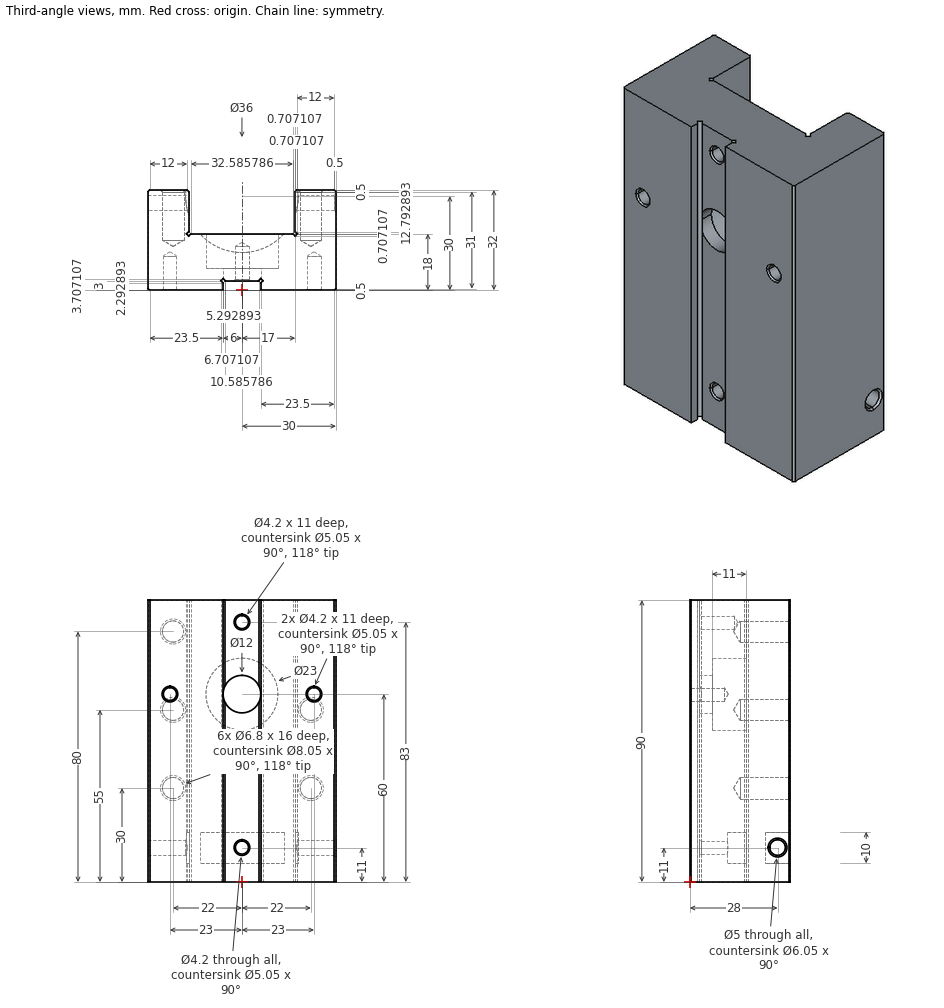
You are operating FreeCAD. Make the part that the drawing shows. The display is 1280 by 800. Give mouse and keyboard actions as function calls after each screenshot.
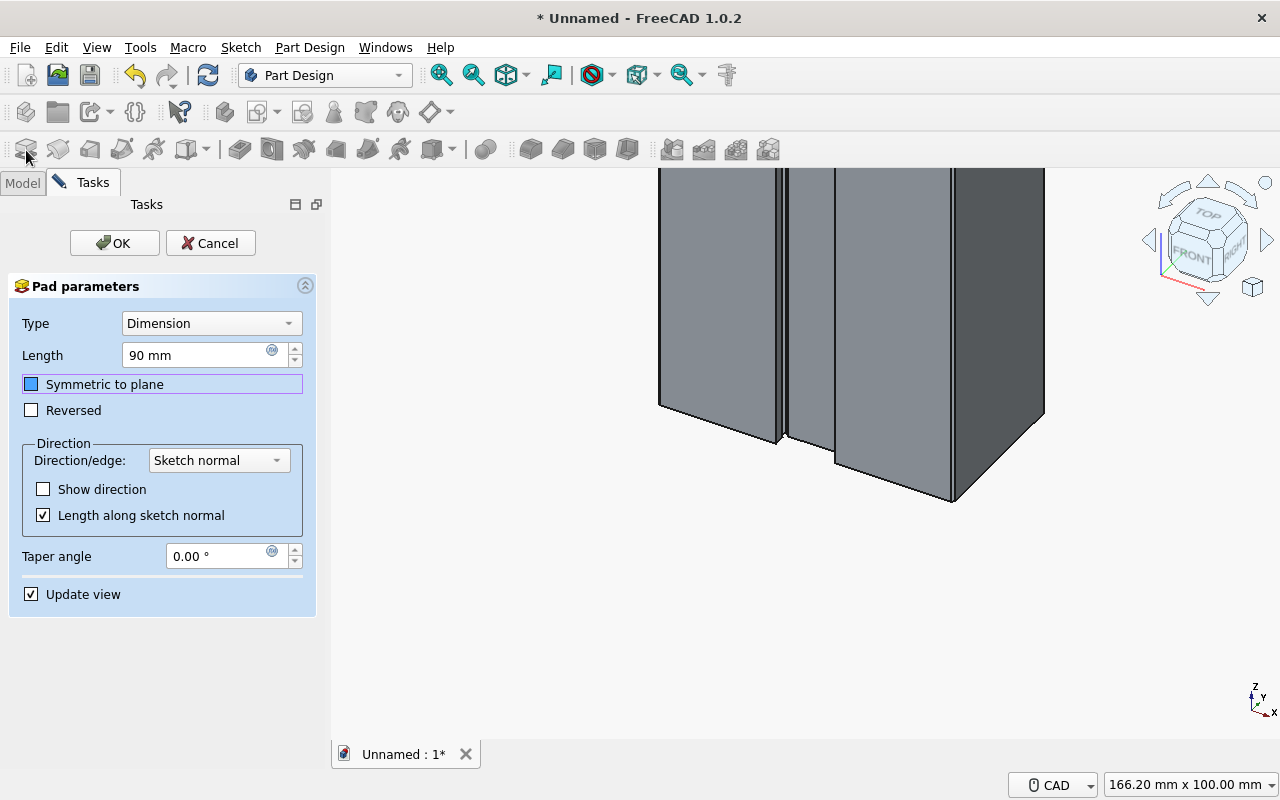
click(115, 243)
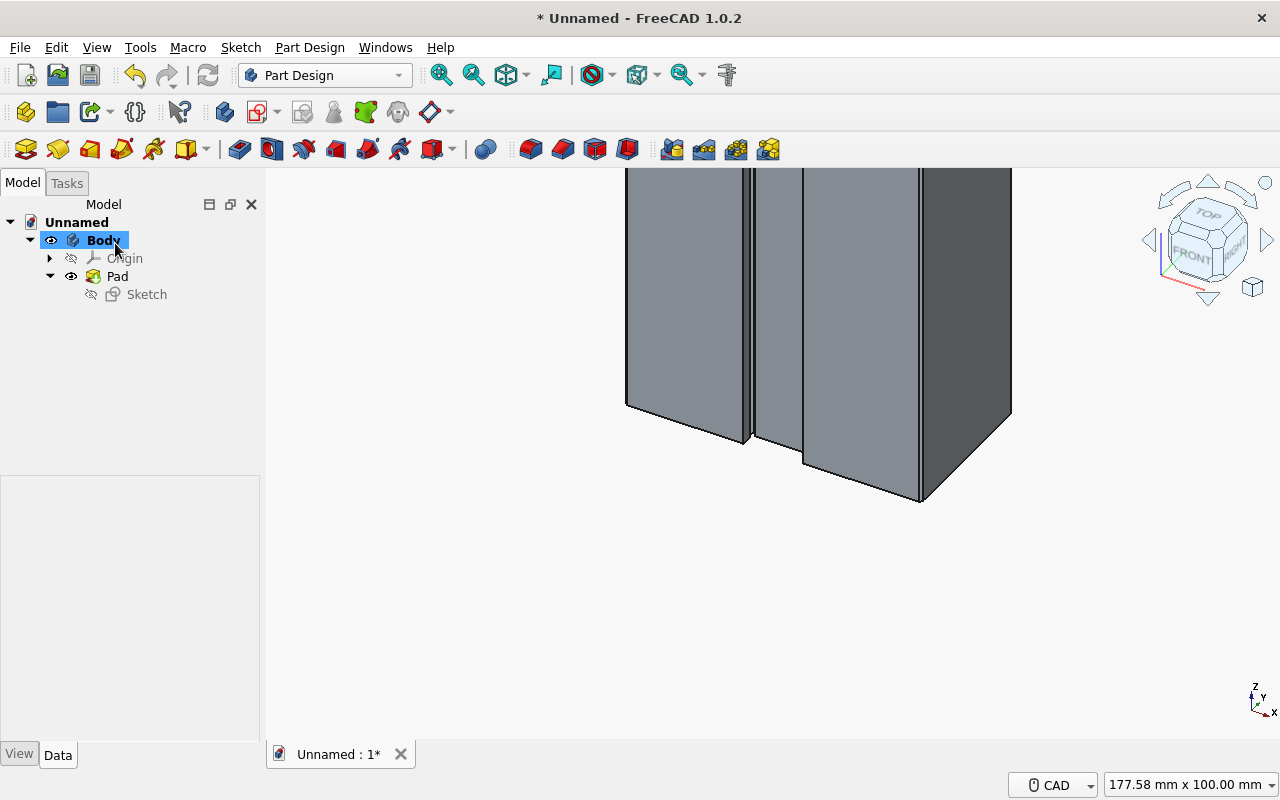
click(442, 76)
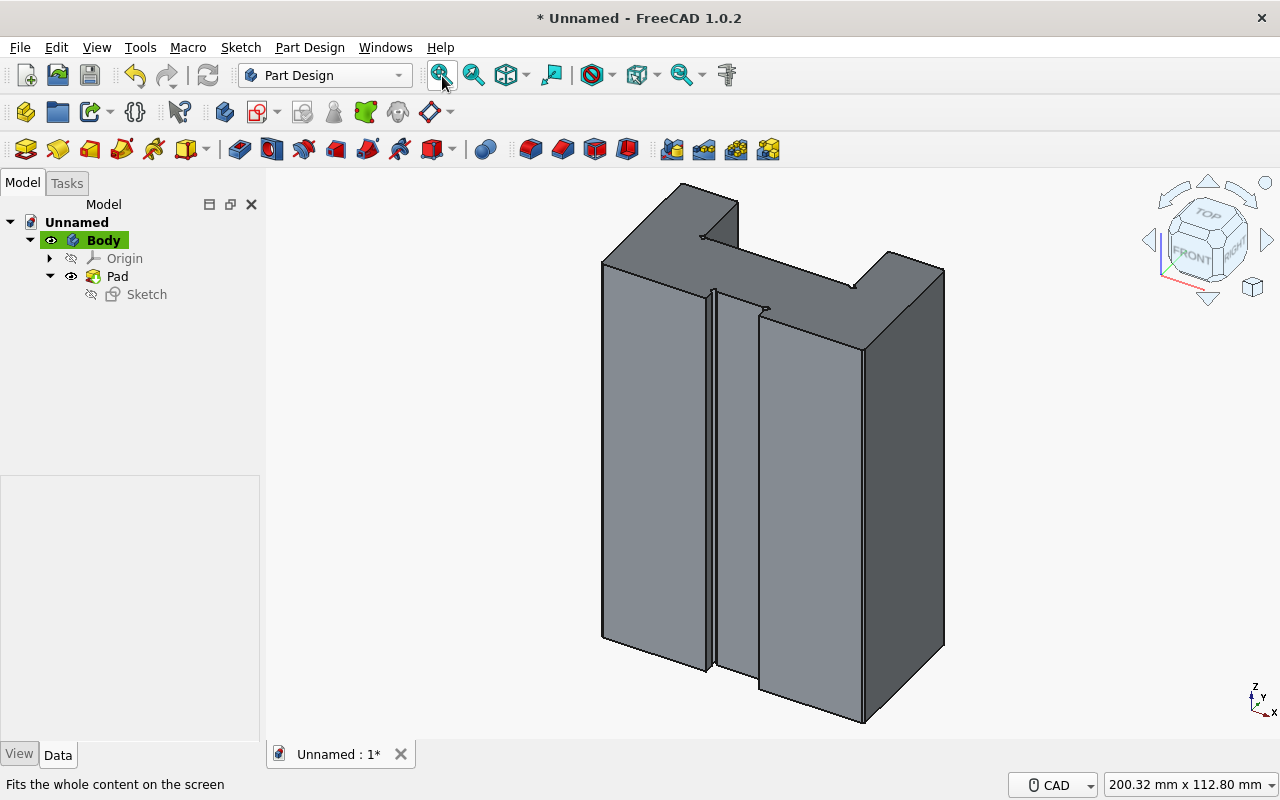
key(4)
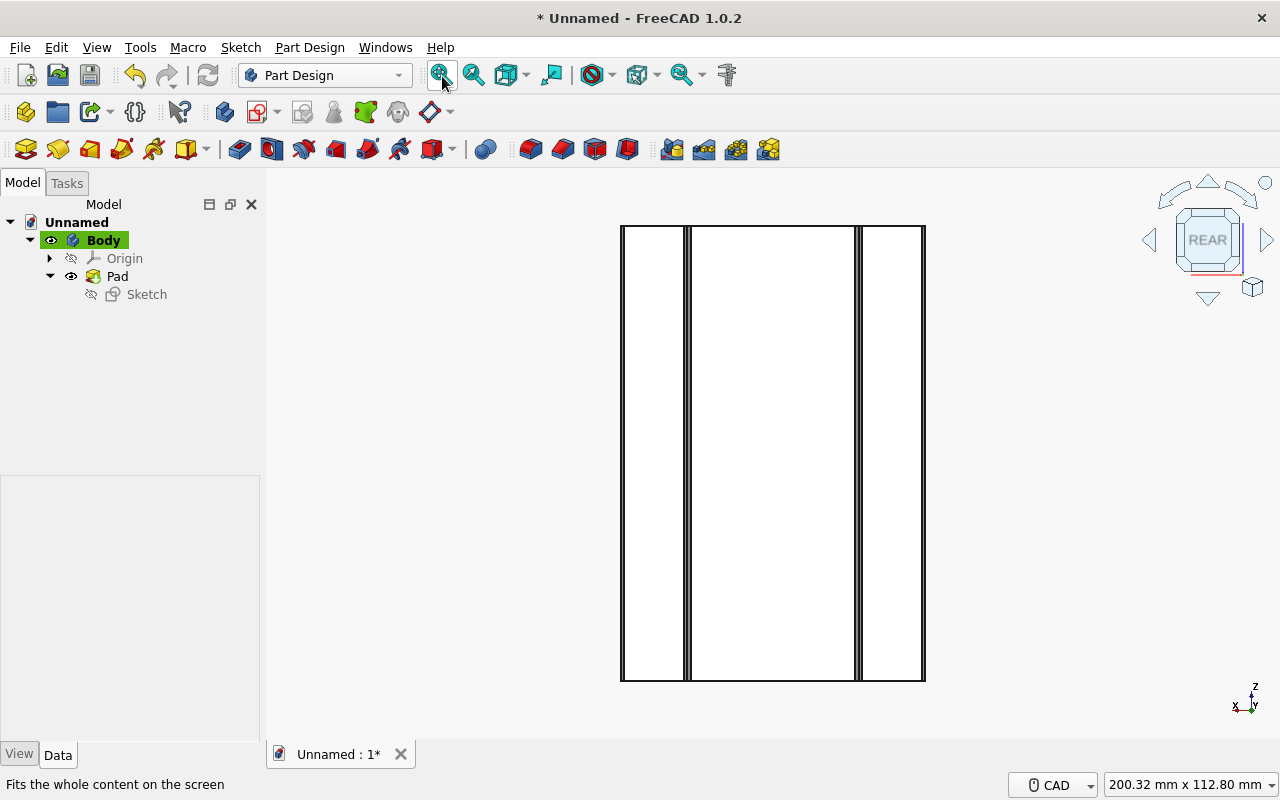
click(773, 322)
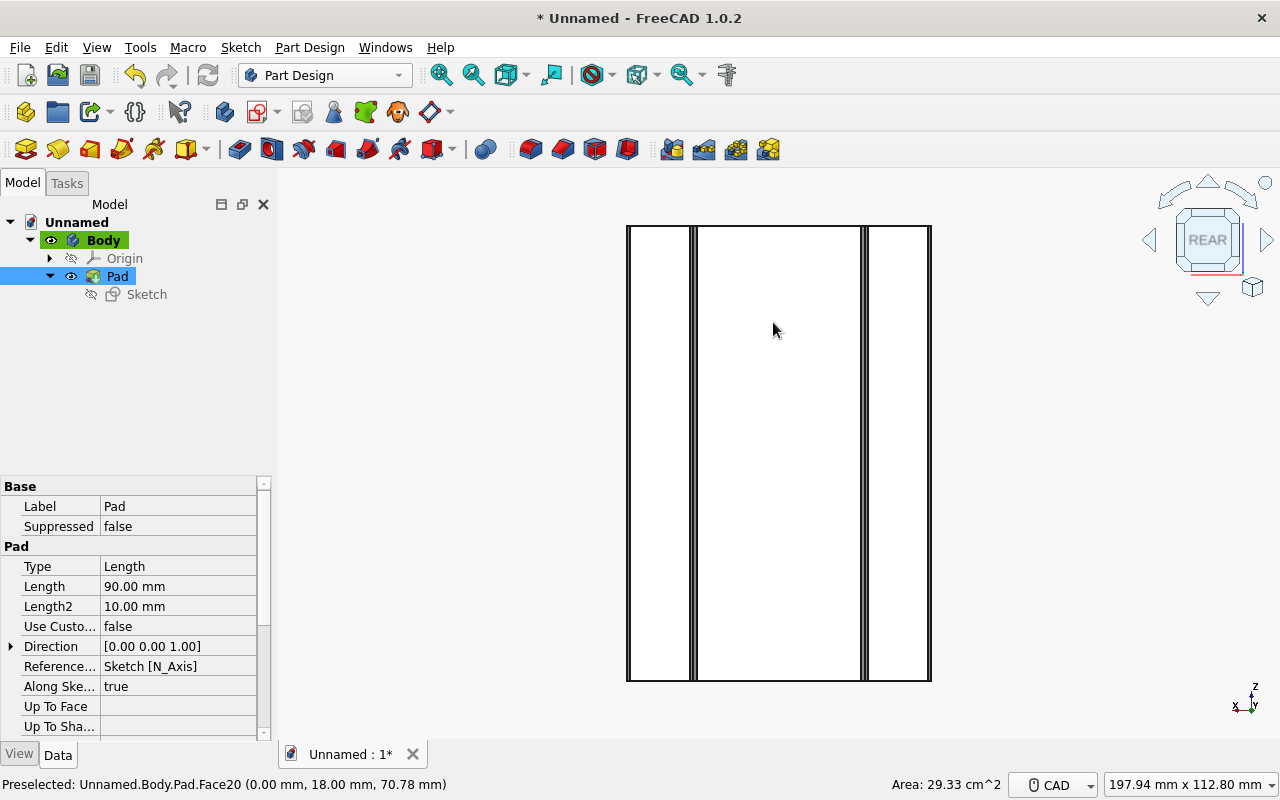
click(258, 112)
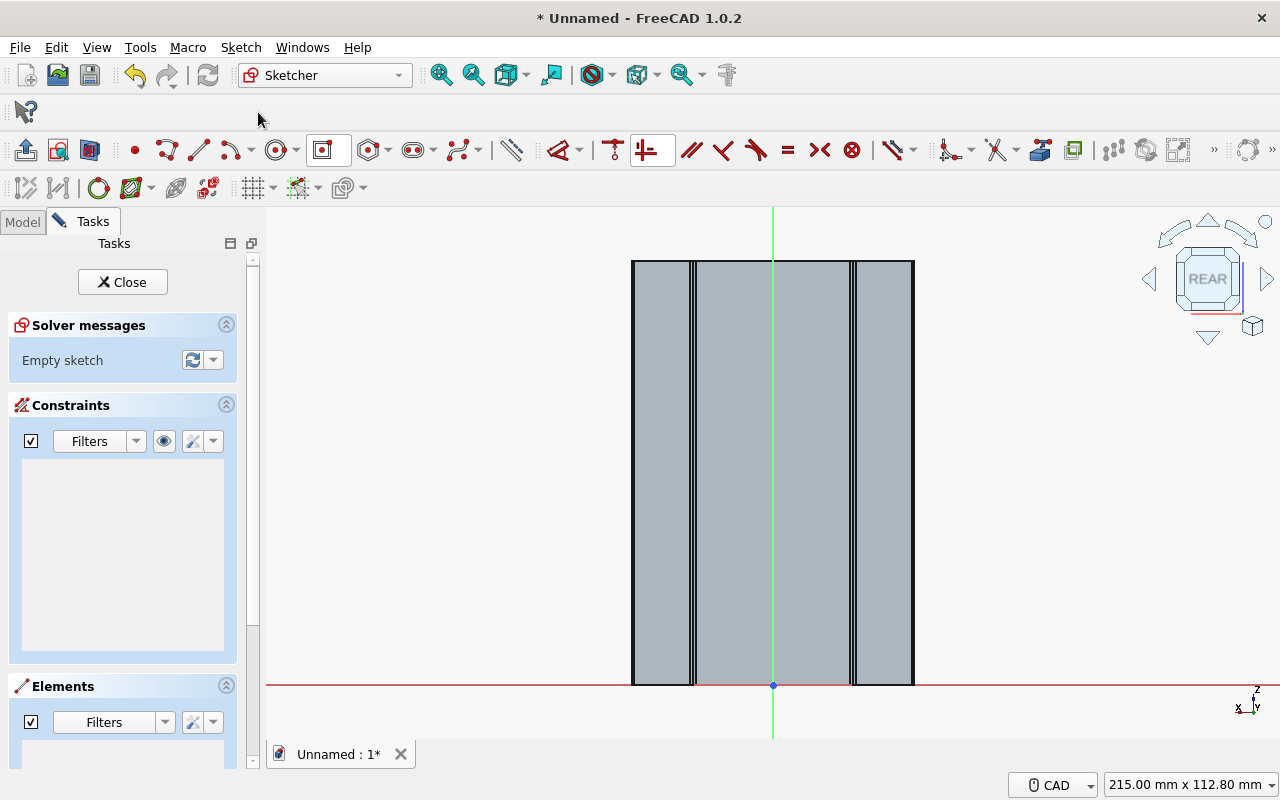
click(90, 150)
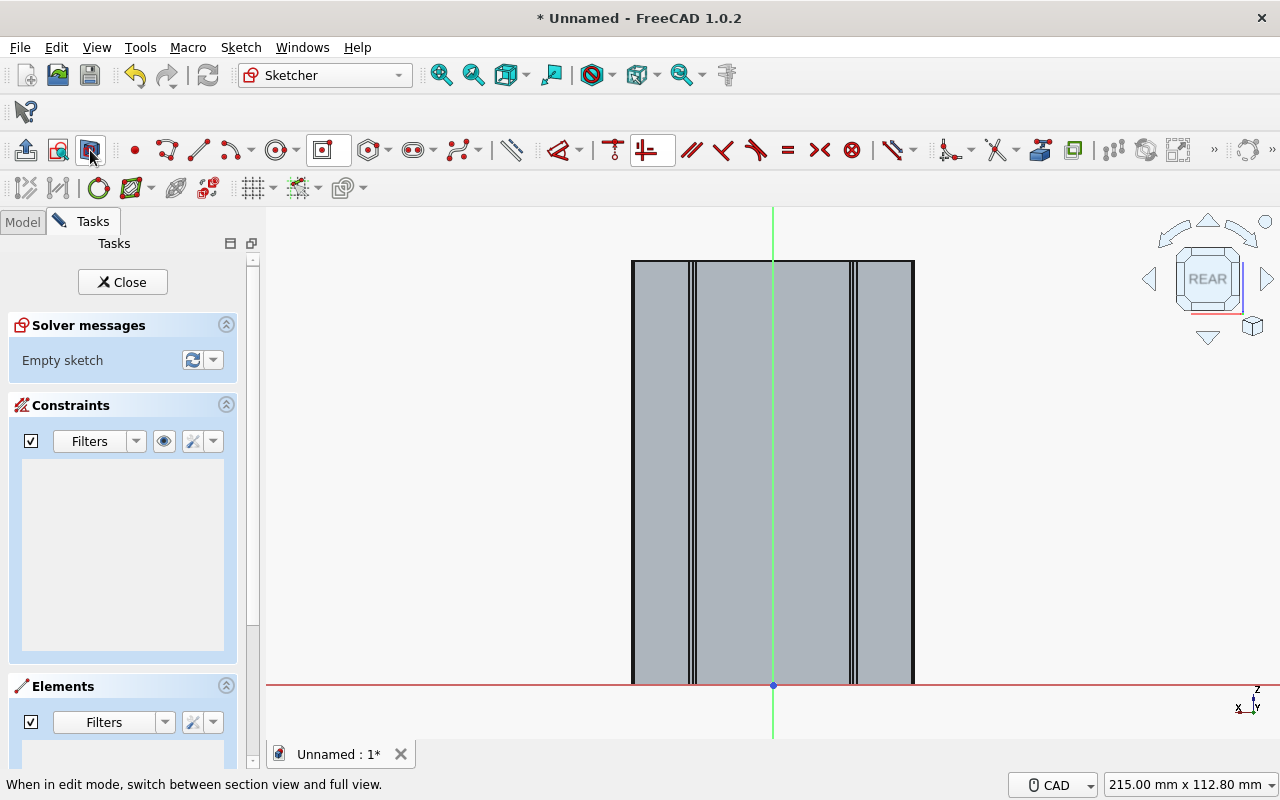
scroll(803, 372, up, 6)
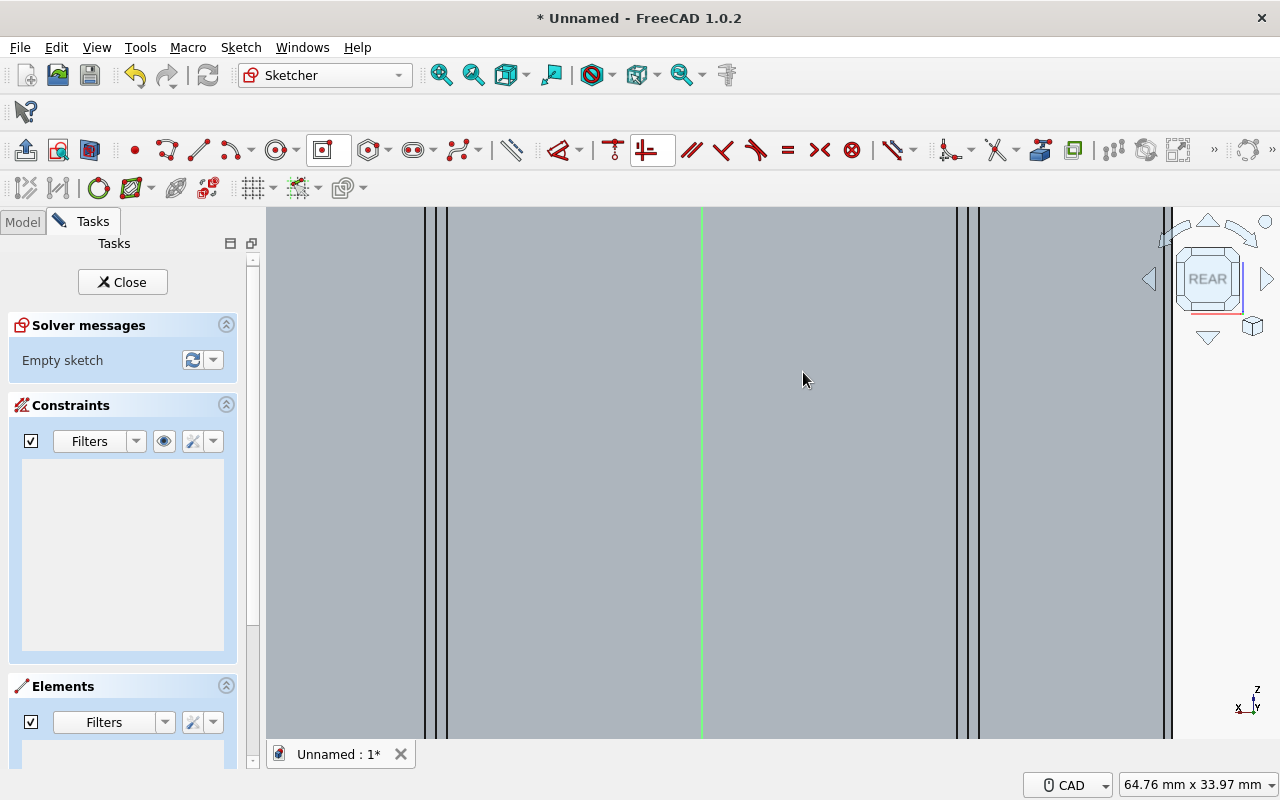
click(276, 150)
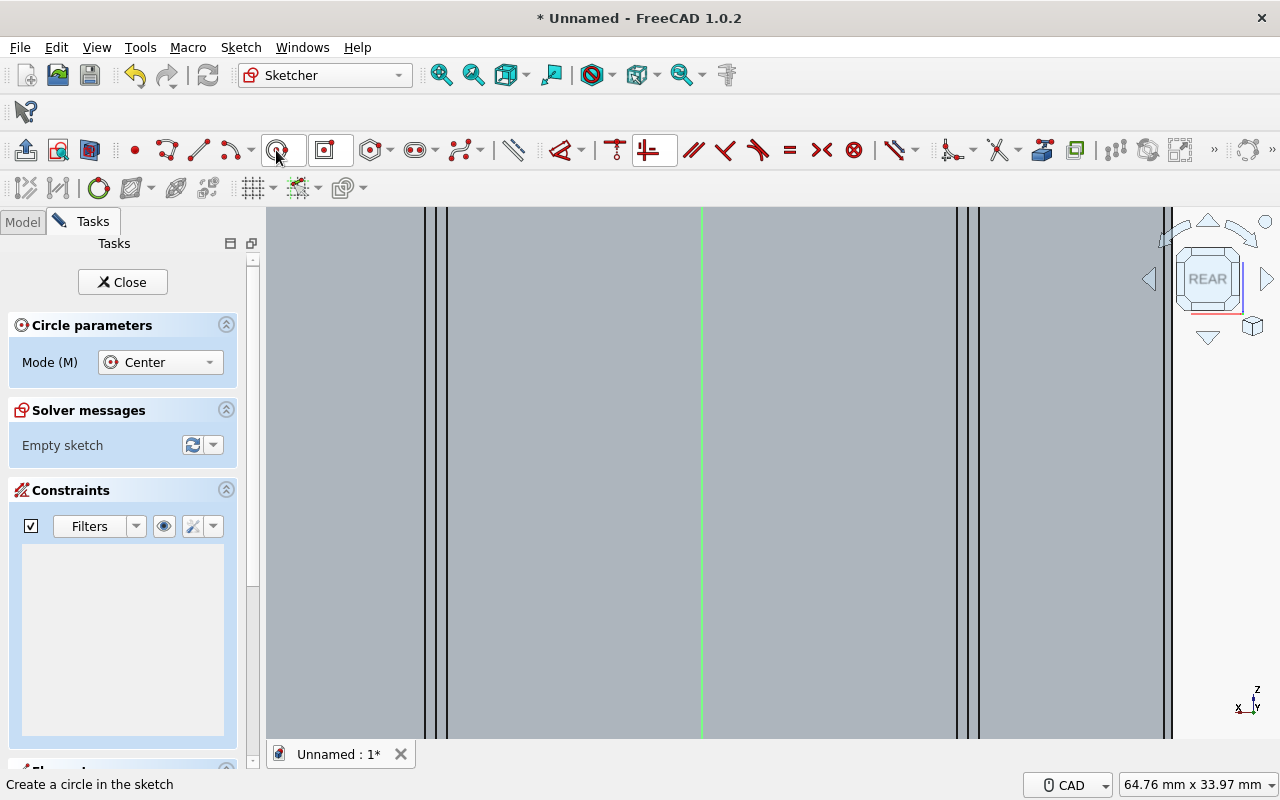
click(702, 472)
move(829, 344)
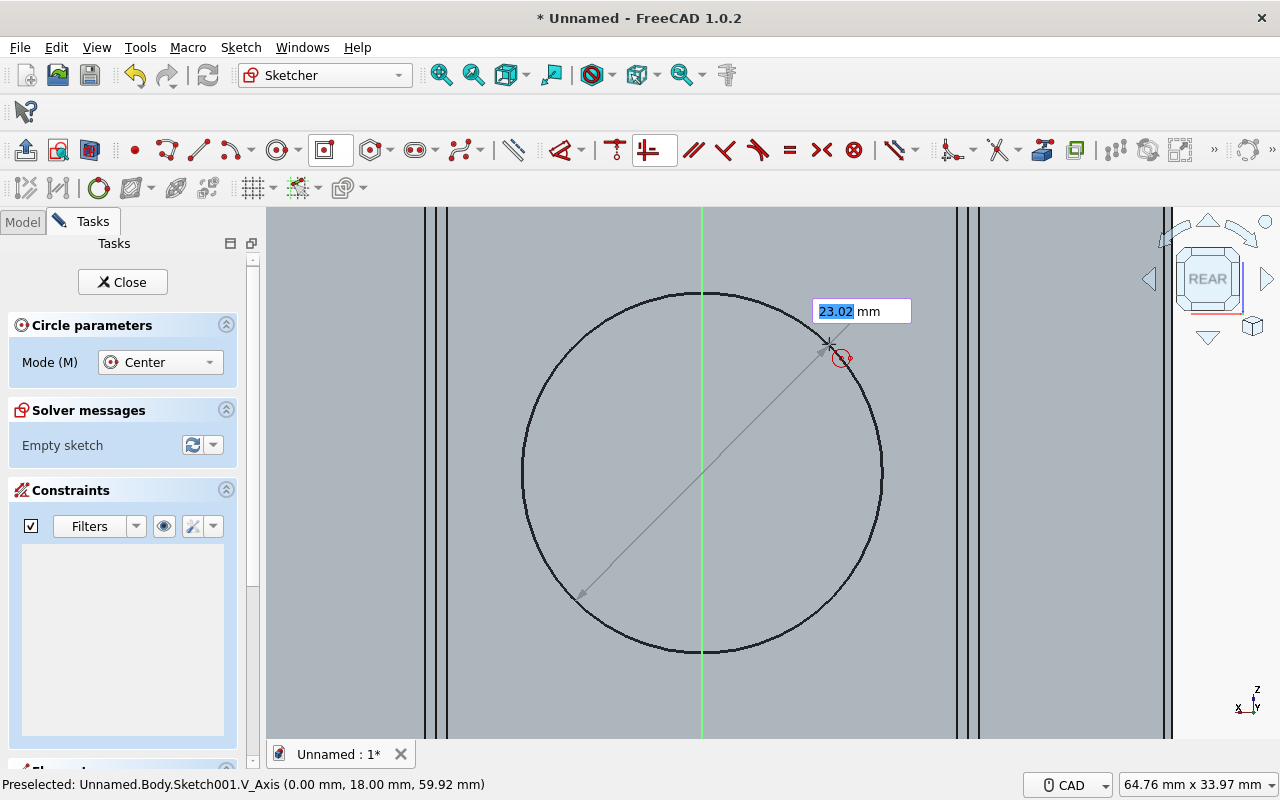
text(23)
key(Return)
key(Escape)